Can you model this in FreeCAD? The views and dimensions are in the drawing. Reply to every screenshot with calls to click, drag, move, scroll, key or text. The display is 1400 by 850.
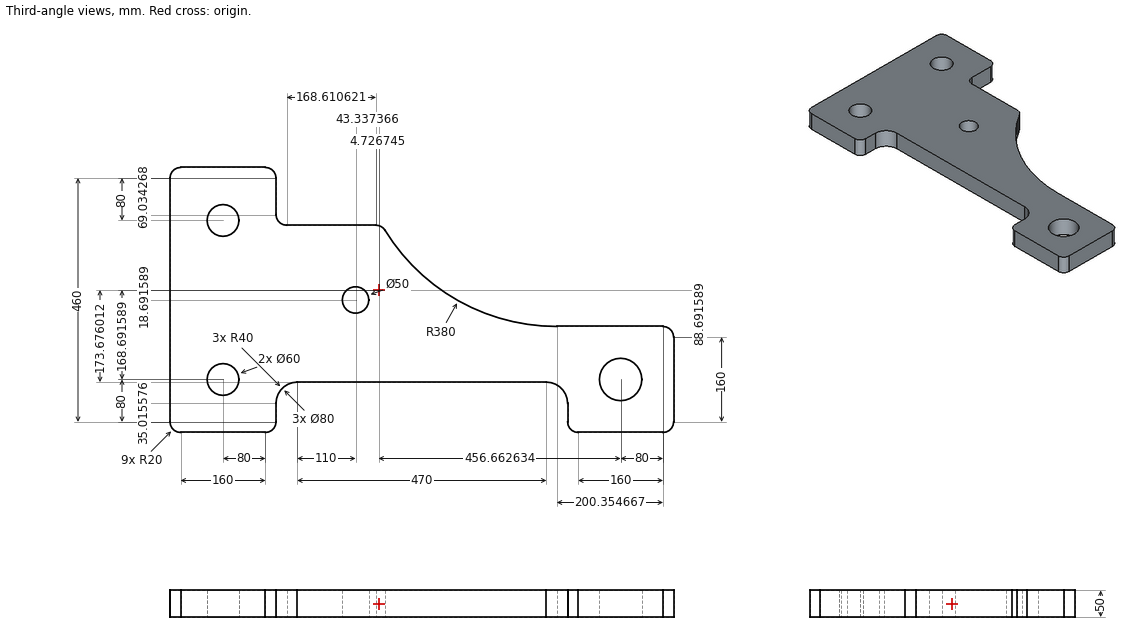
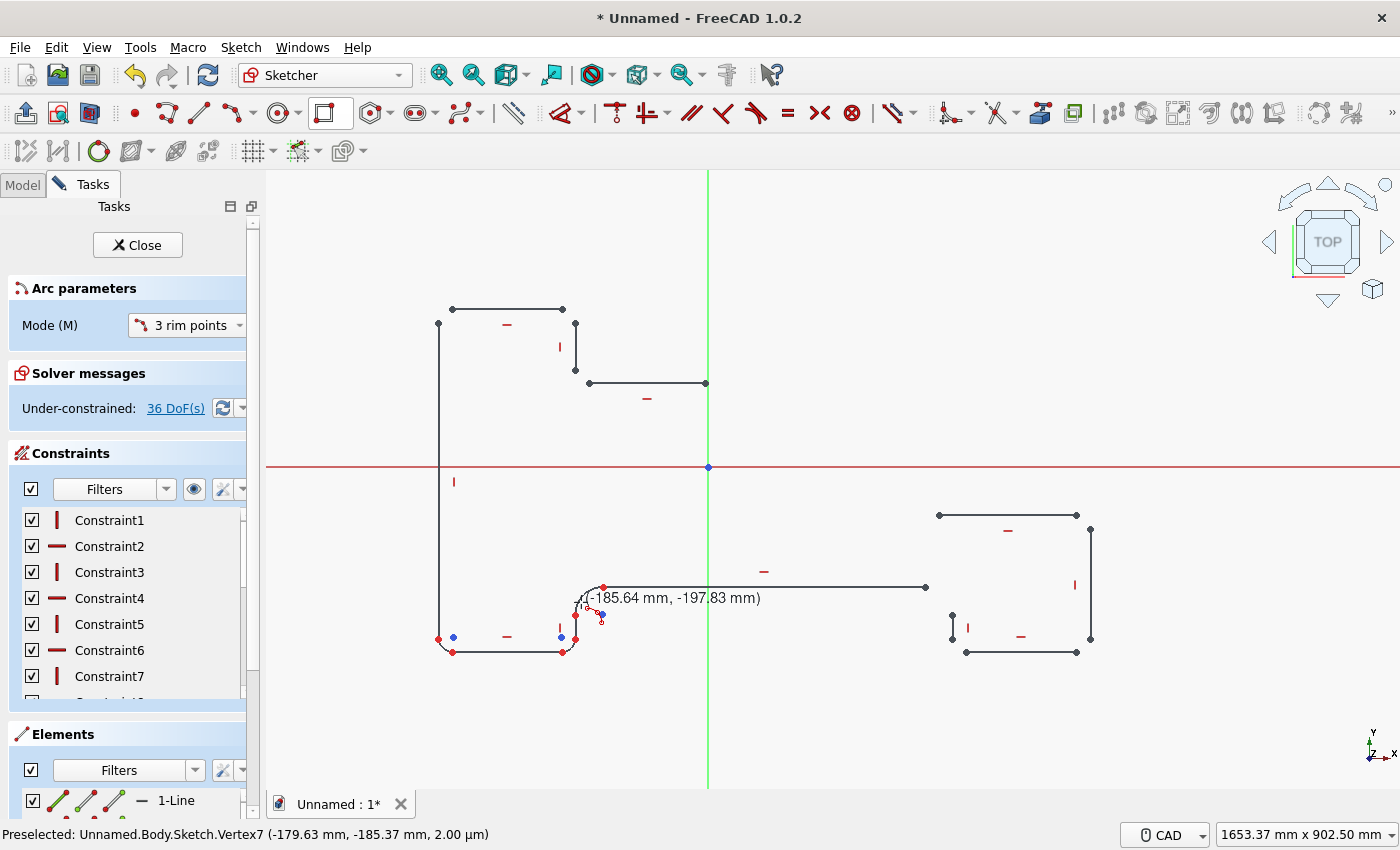
click(926, 587)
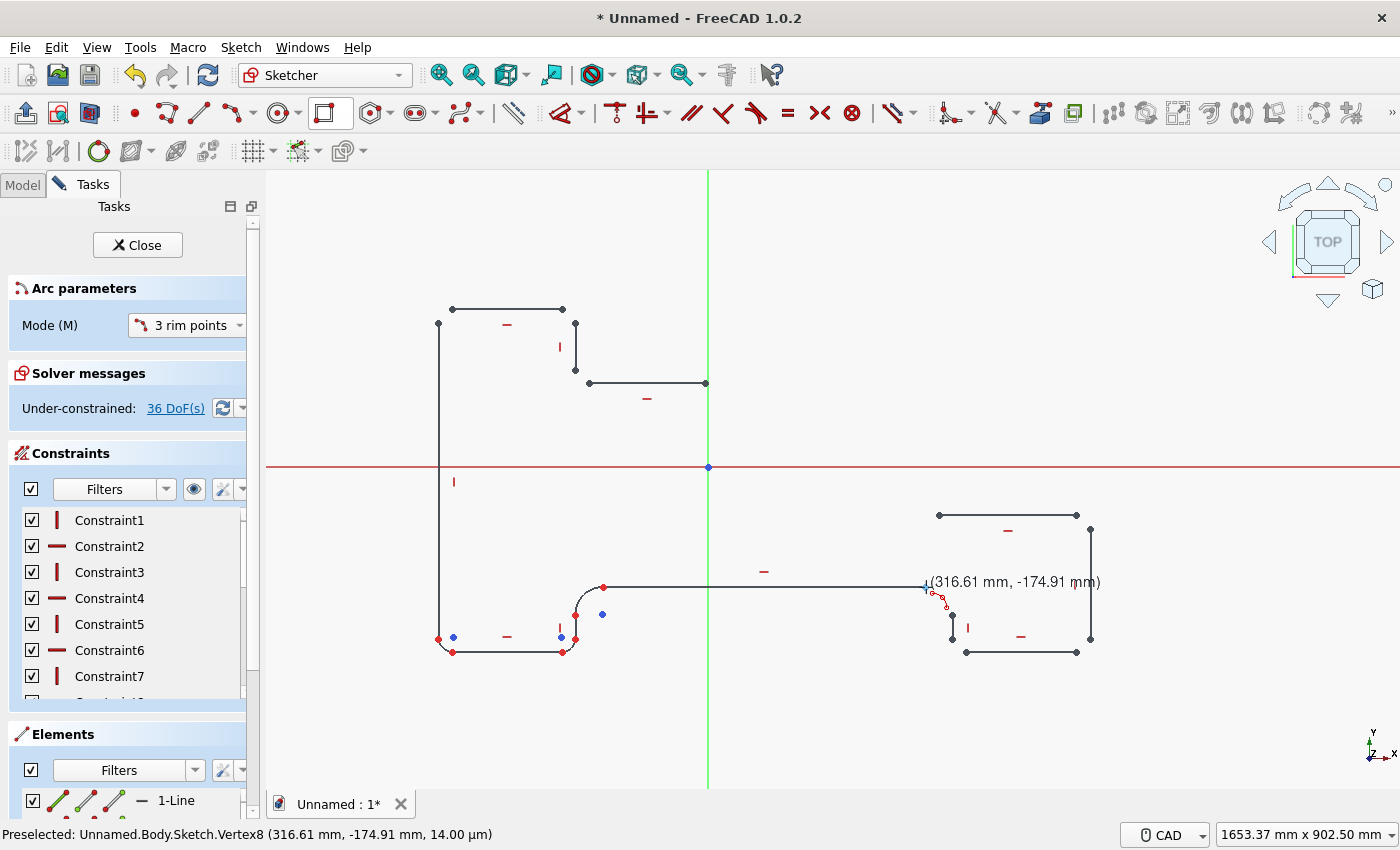
scroll(953, 614, up, 2)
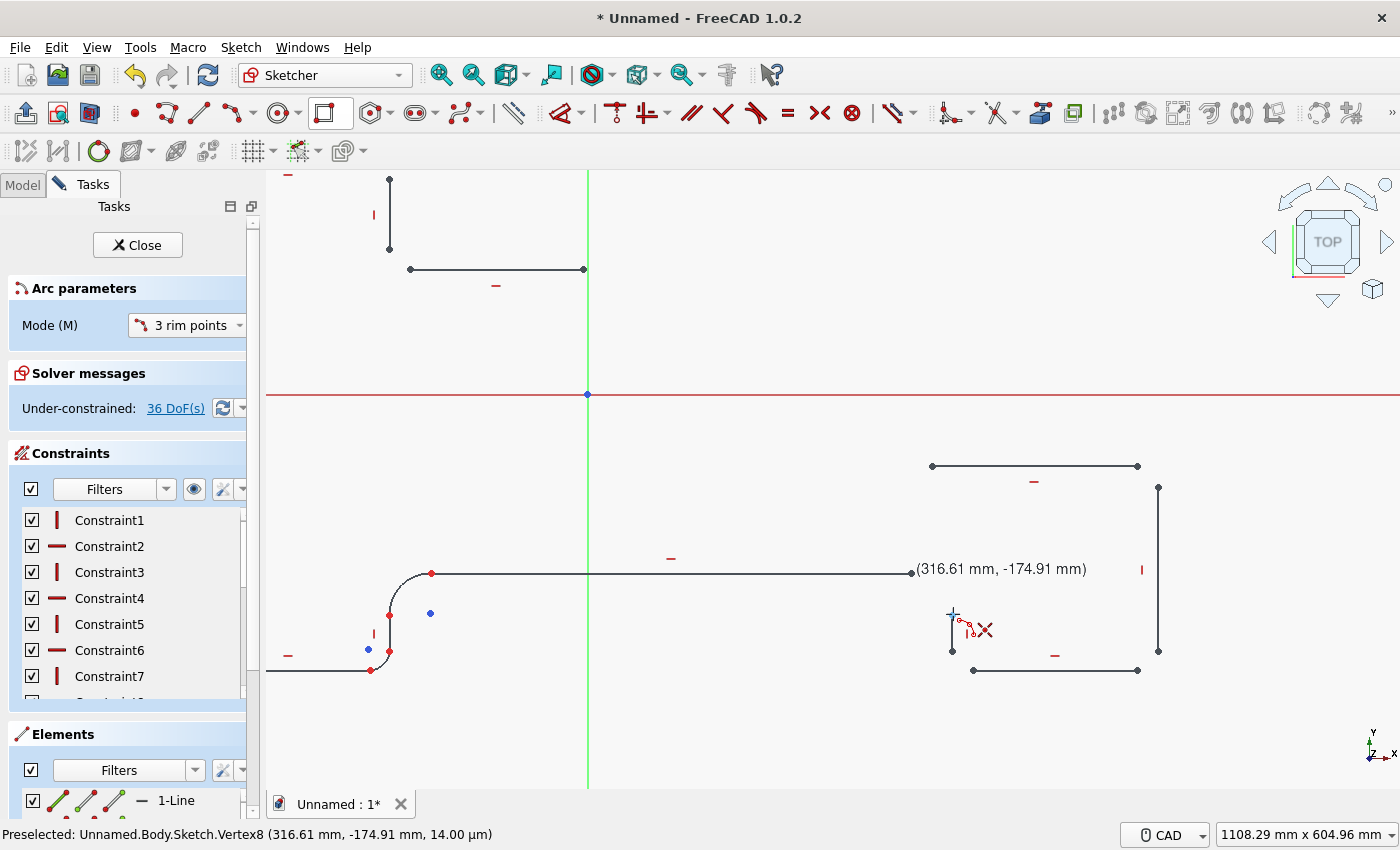
click(952, 615)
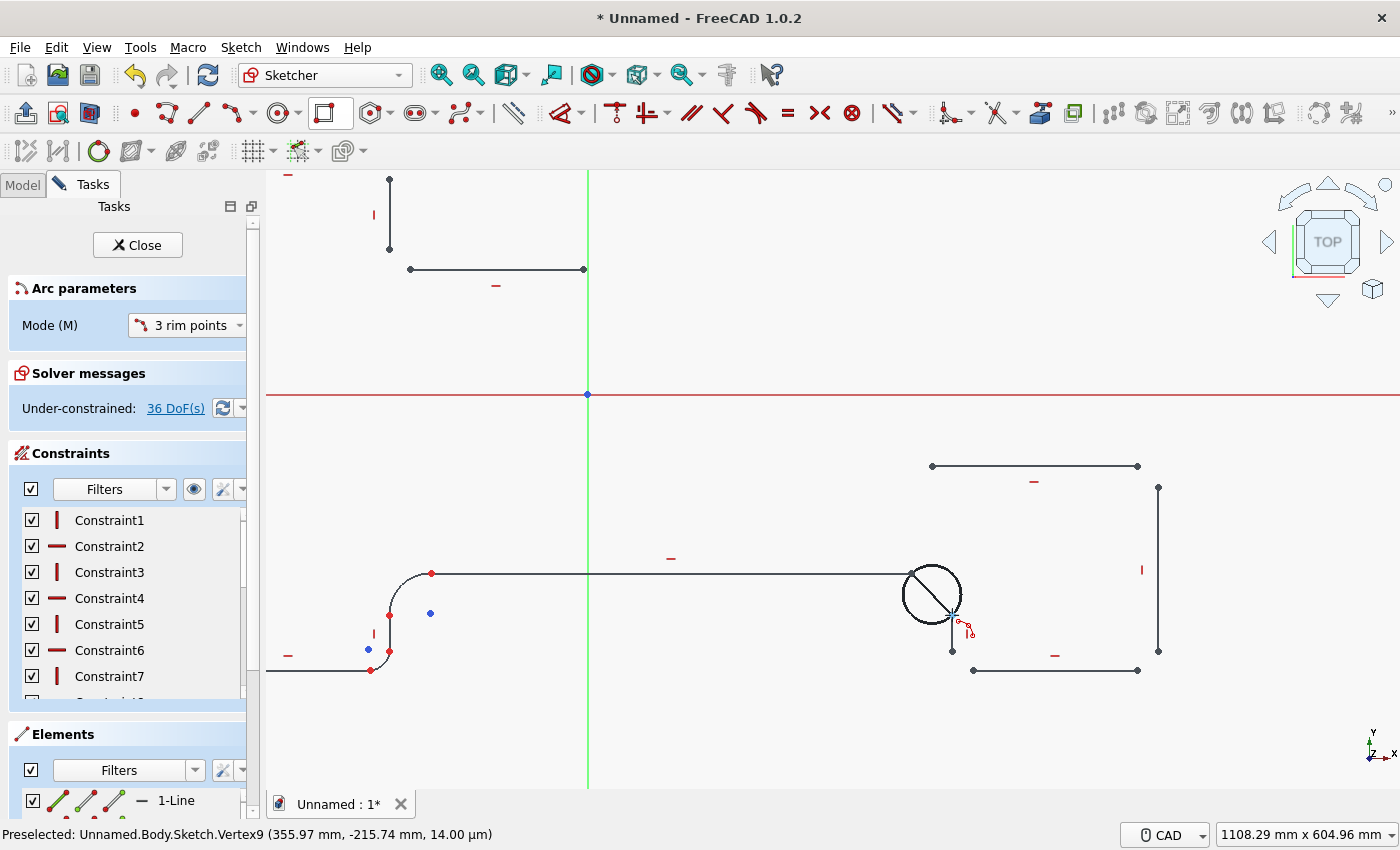
scroll(941, 584, up, 2)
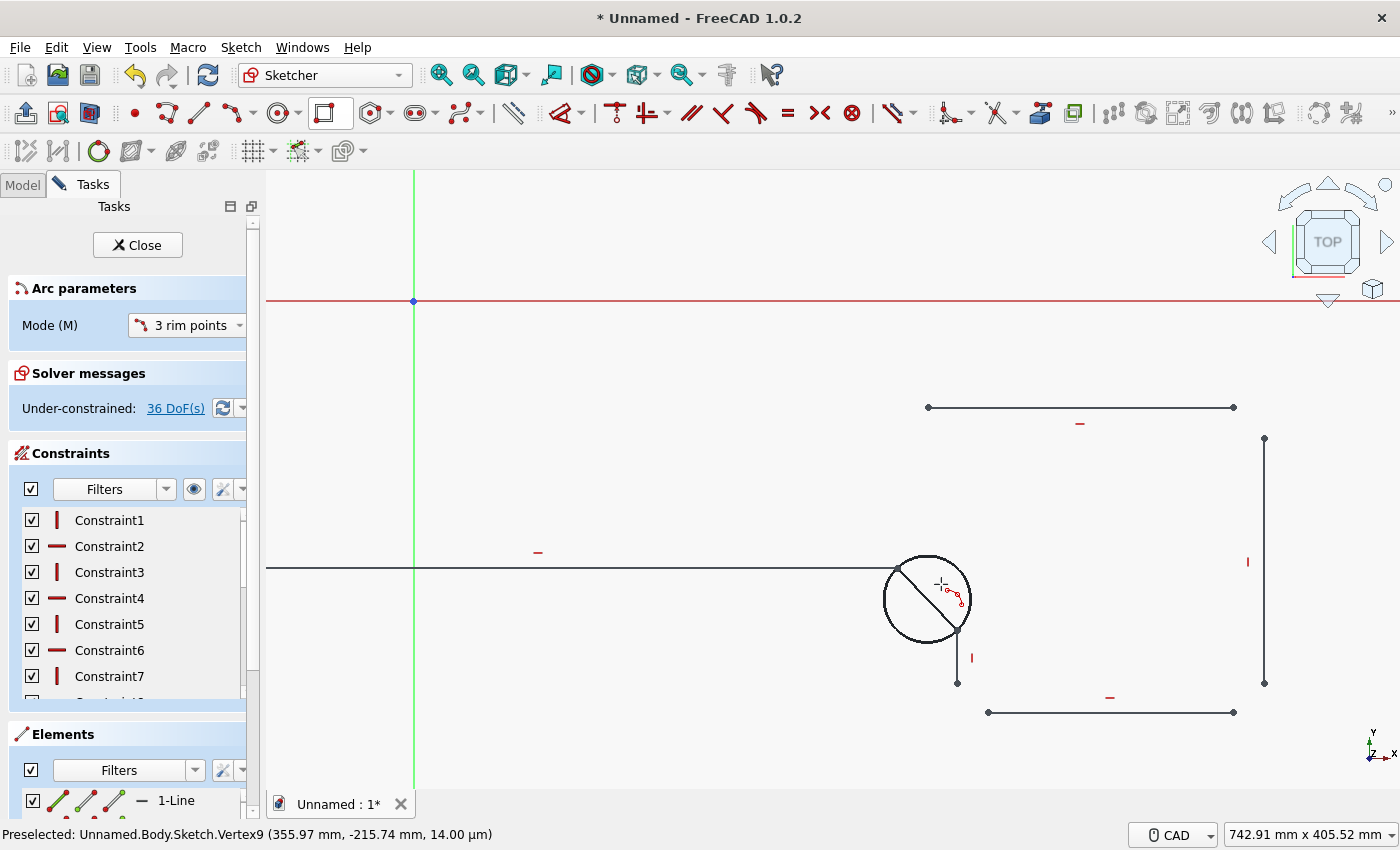
click(941, 584)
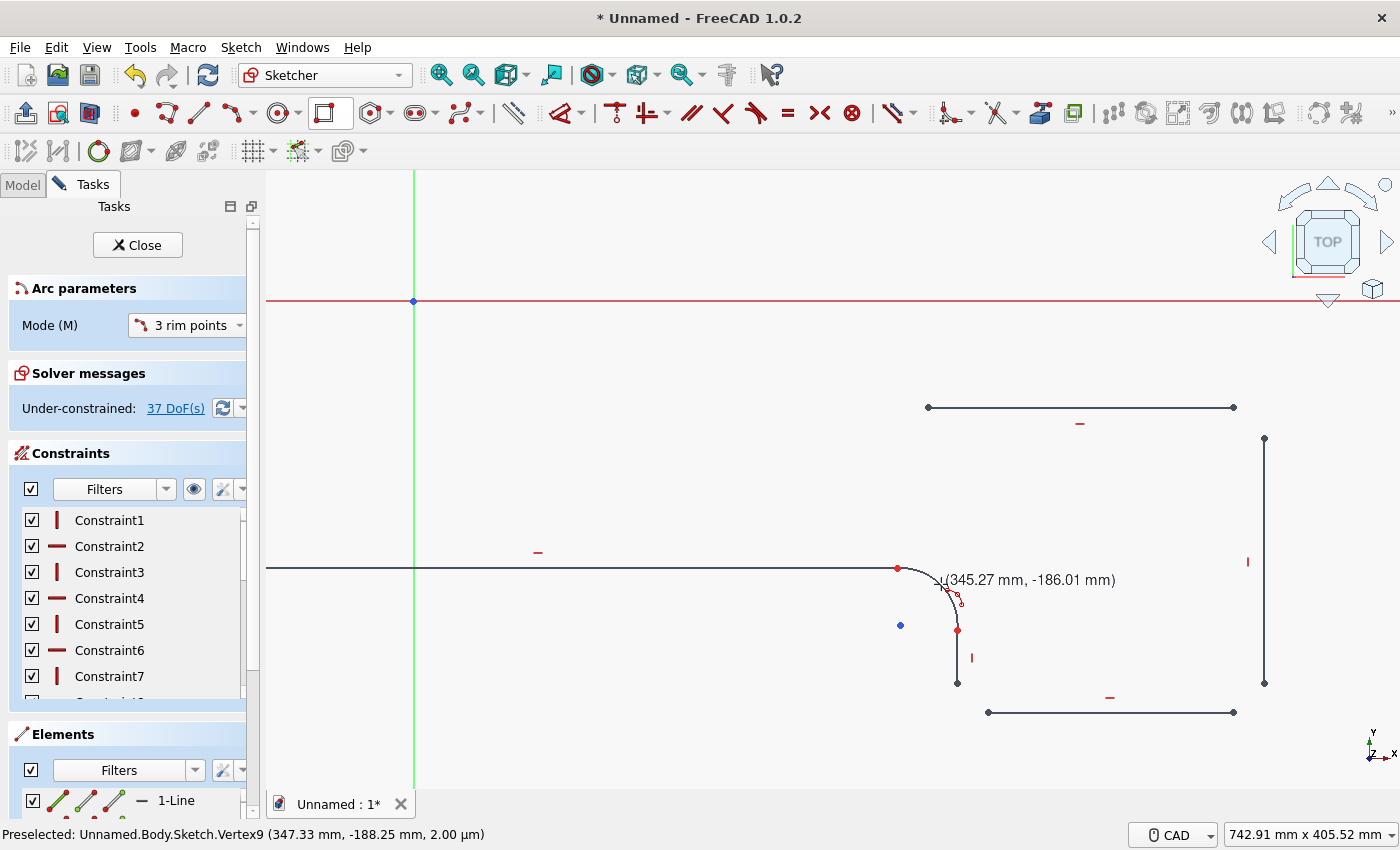
click(957, 684)
click(988, 713)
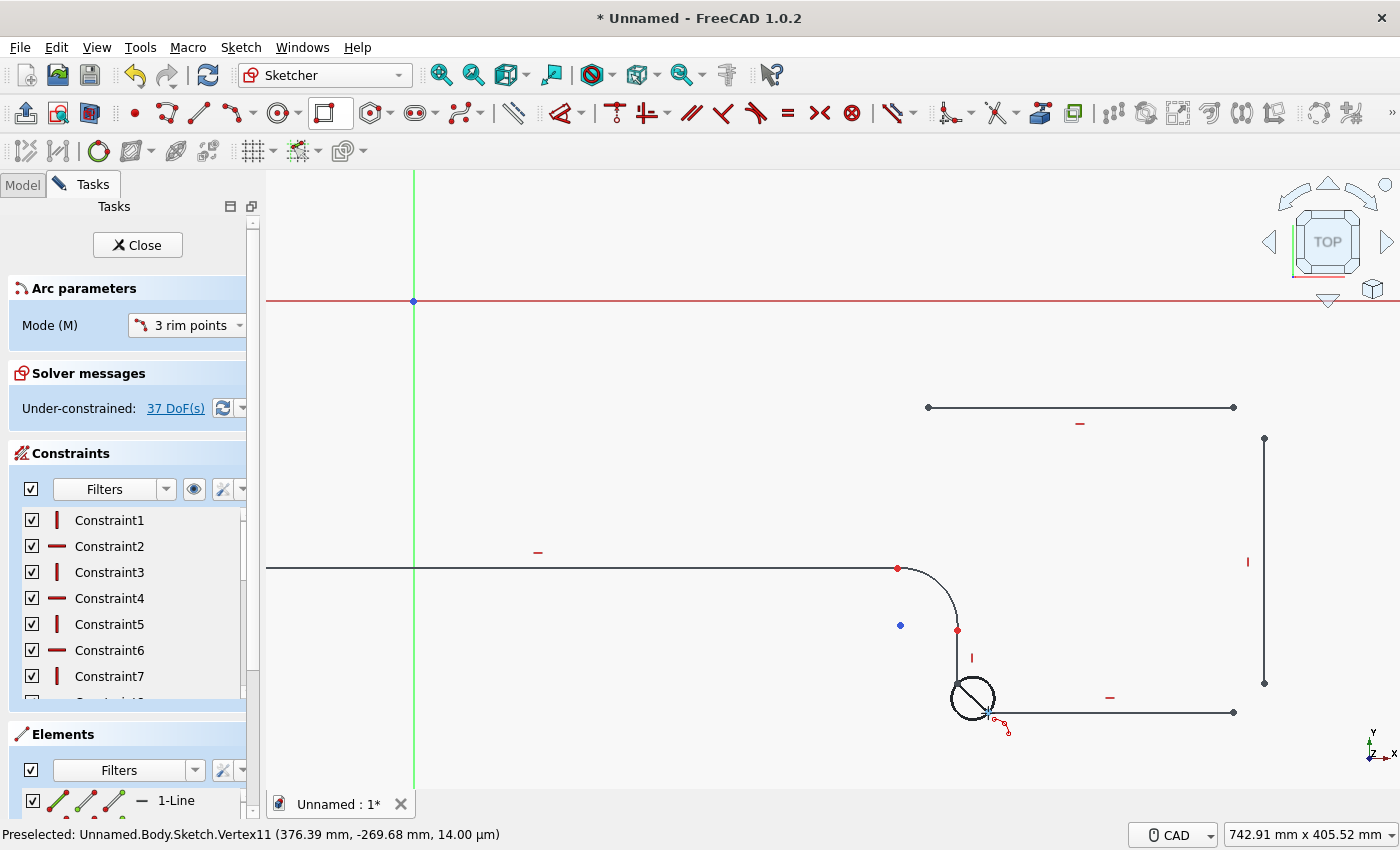
scroll(967, 702, up, 3)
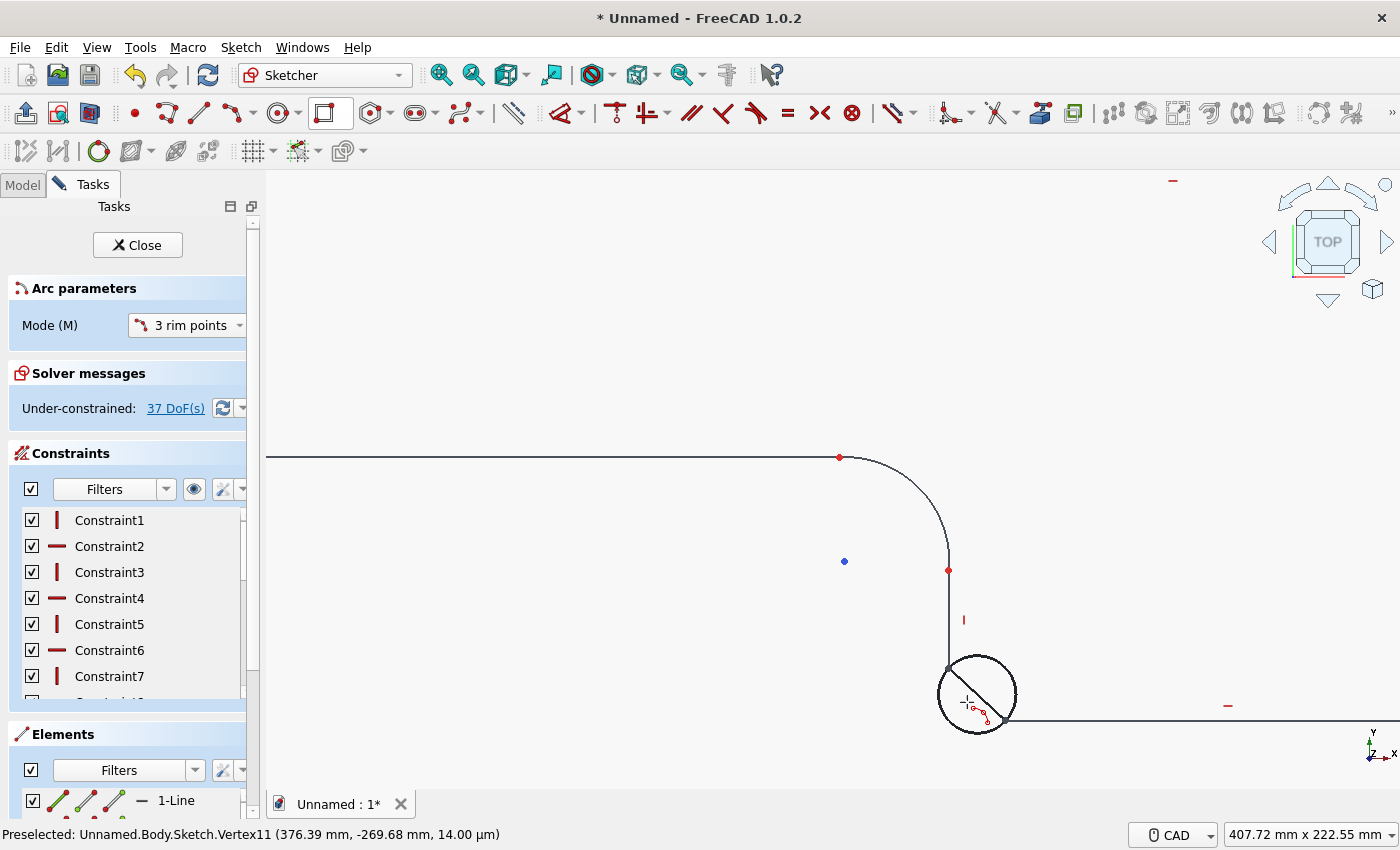
click(967, 702)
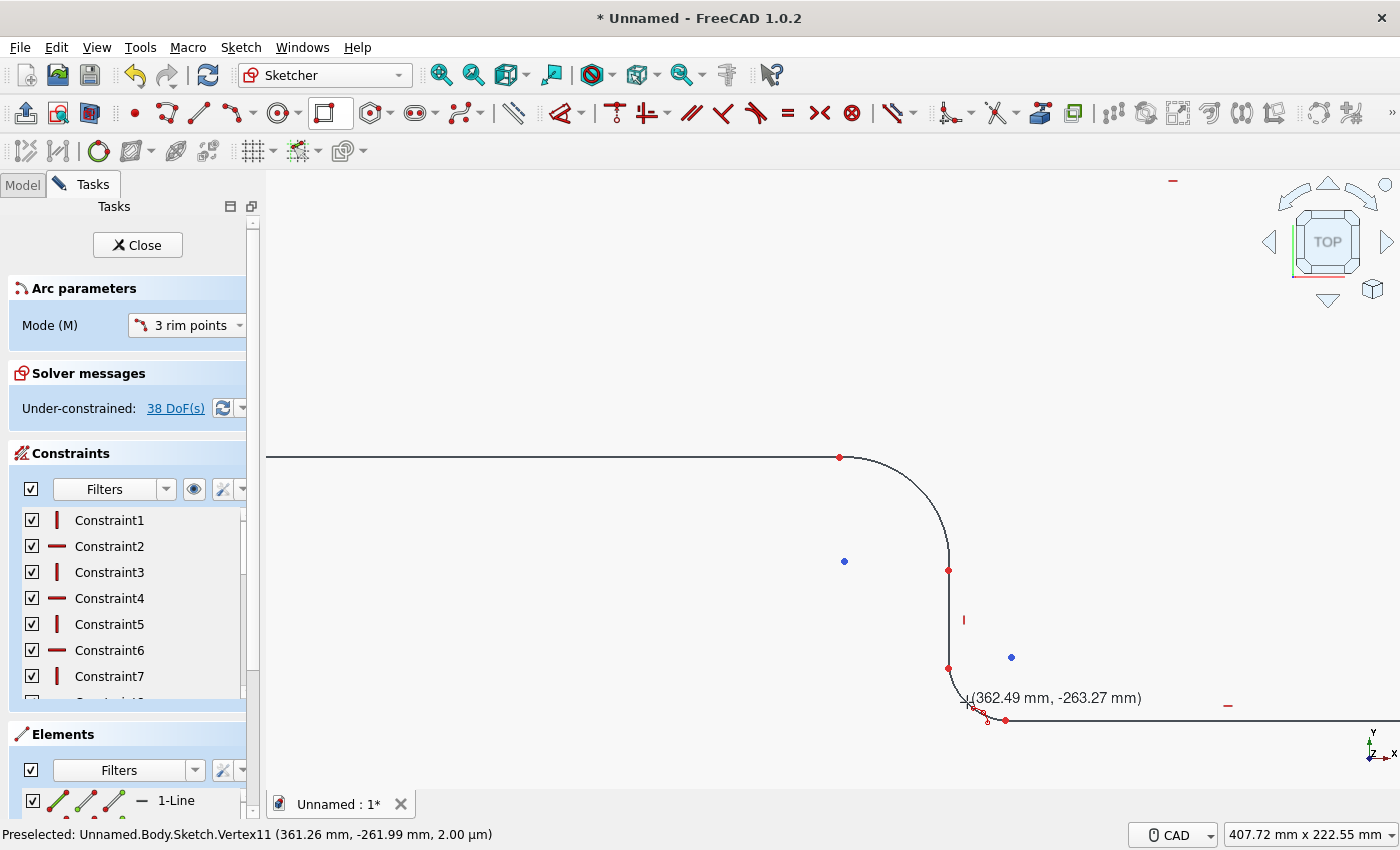
scroll(954, 629, down, 7)